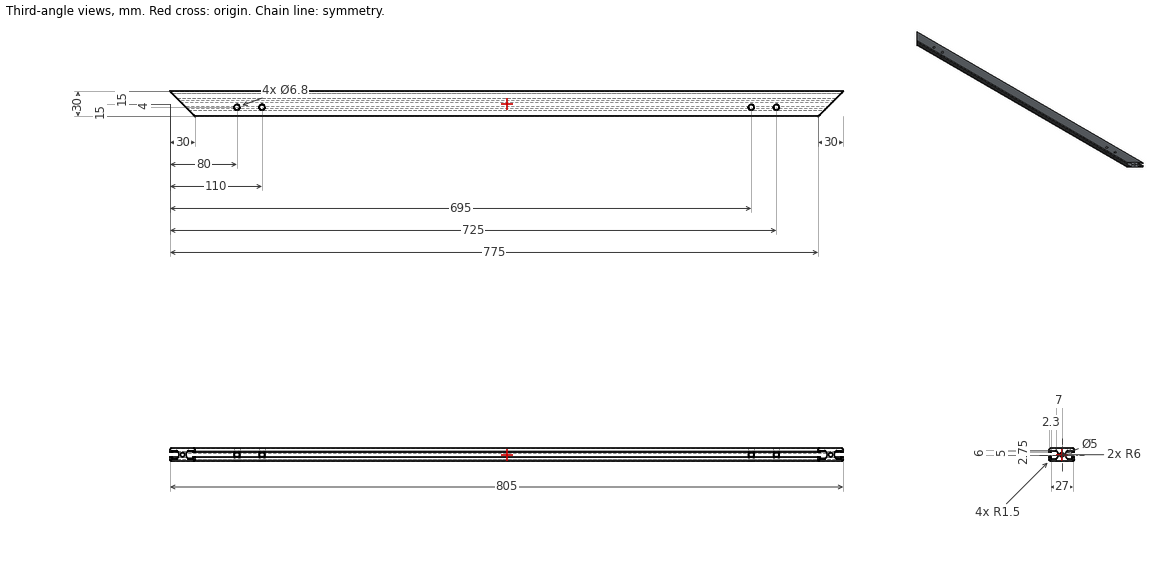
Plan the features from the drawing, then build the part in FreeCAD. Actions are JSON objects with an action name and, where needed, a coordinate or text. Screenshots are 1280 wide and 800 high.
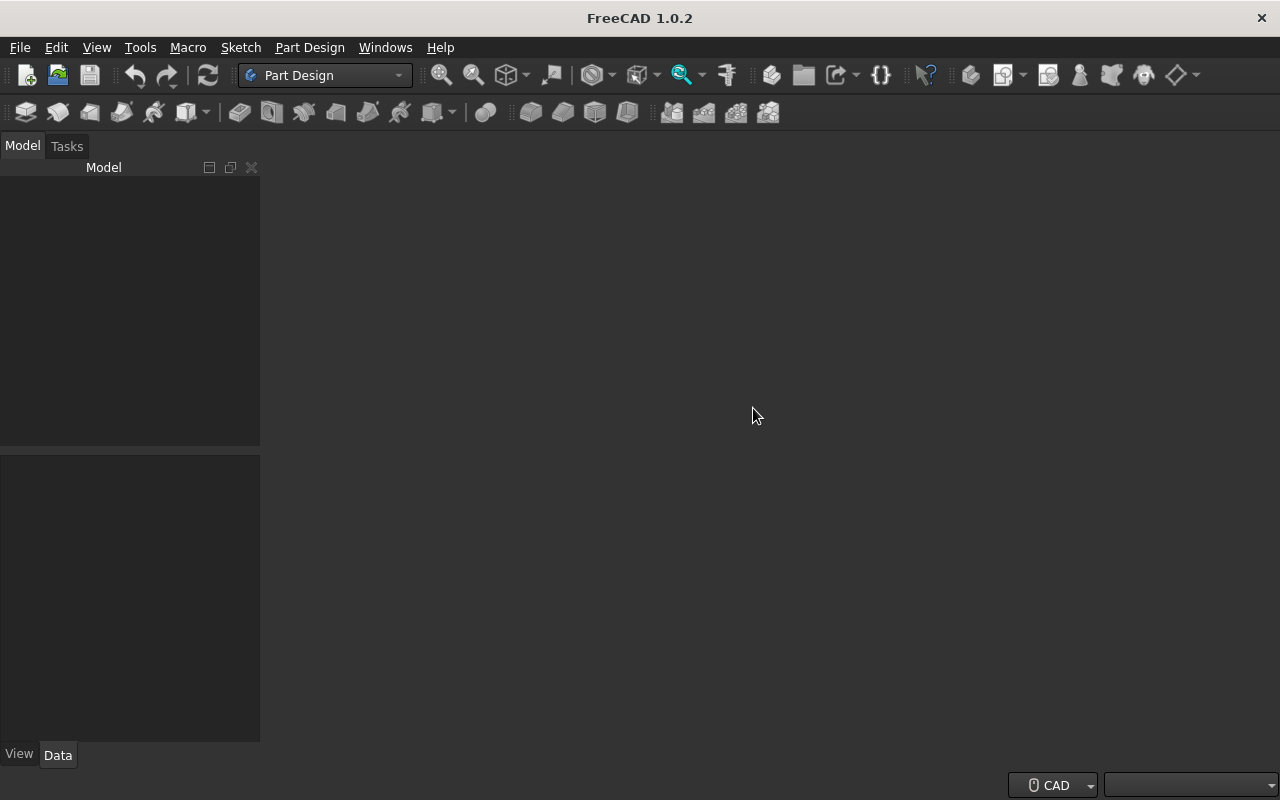
{"action": "left_click", "coordinate": [26, 76]}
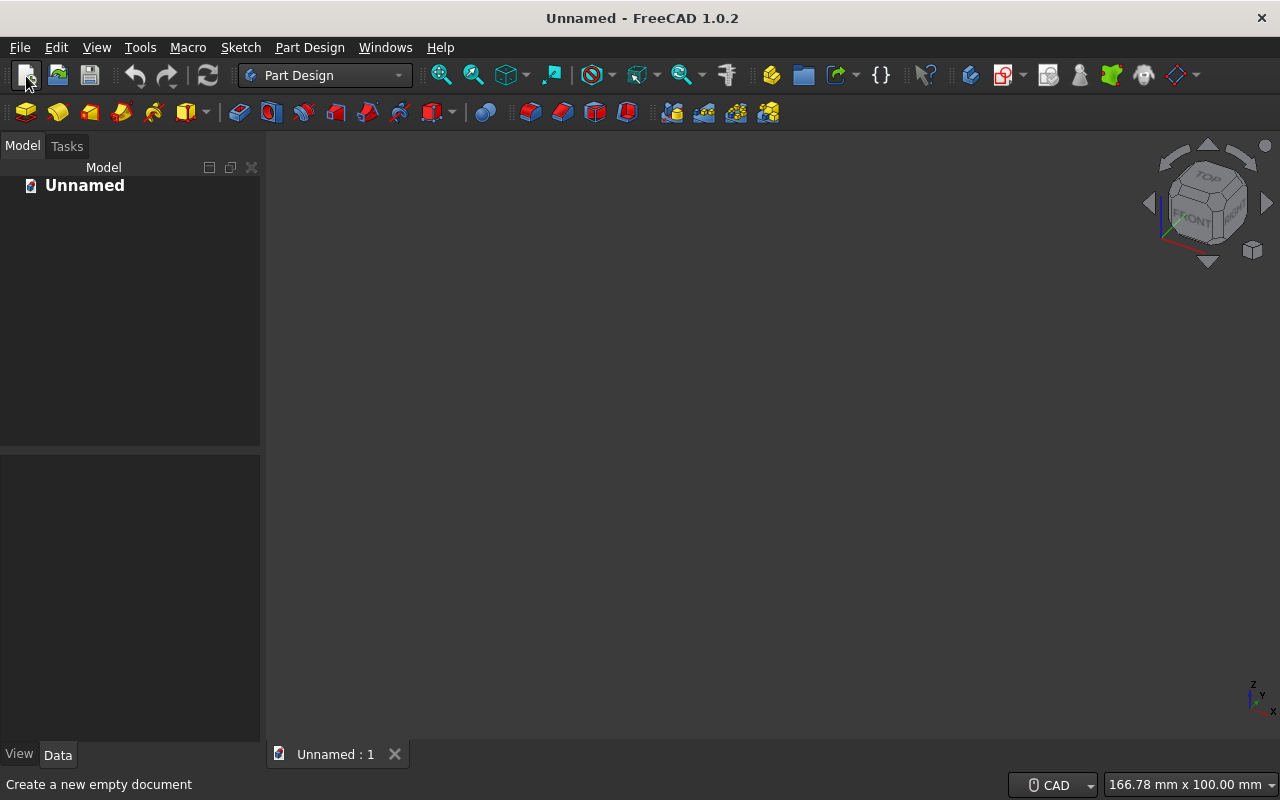
{"action": "left_click", "coordinate": [972, 76]}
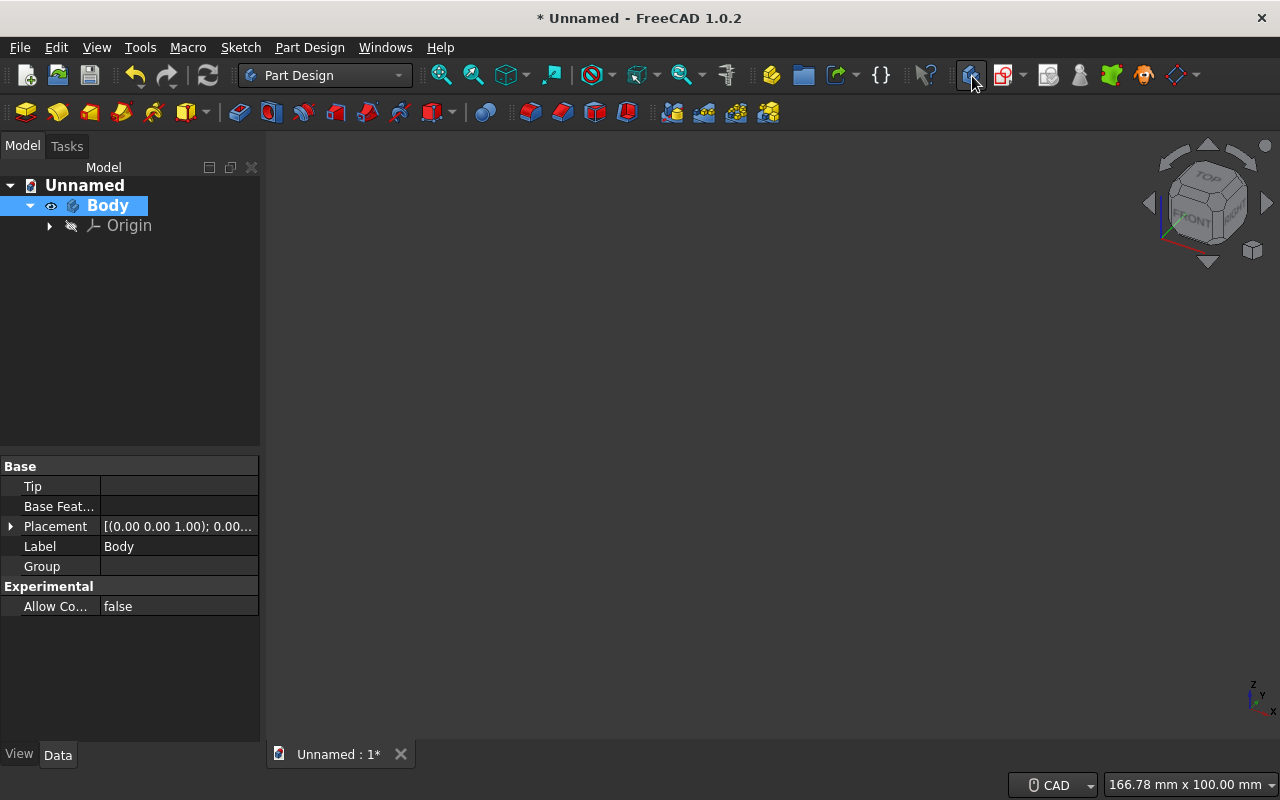
{"action": "left_click", "coordinate": [50, 226]}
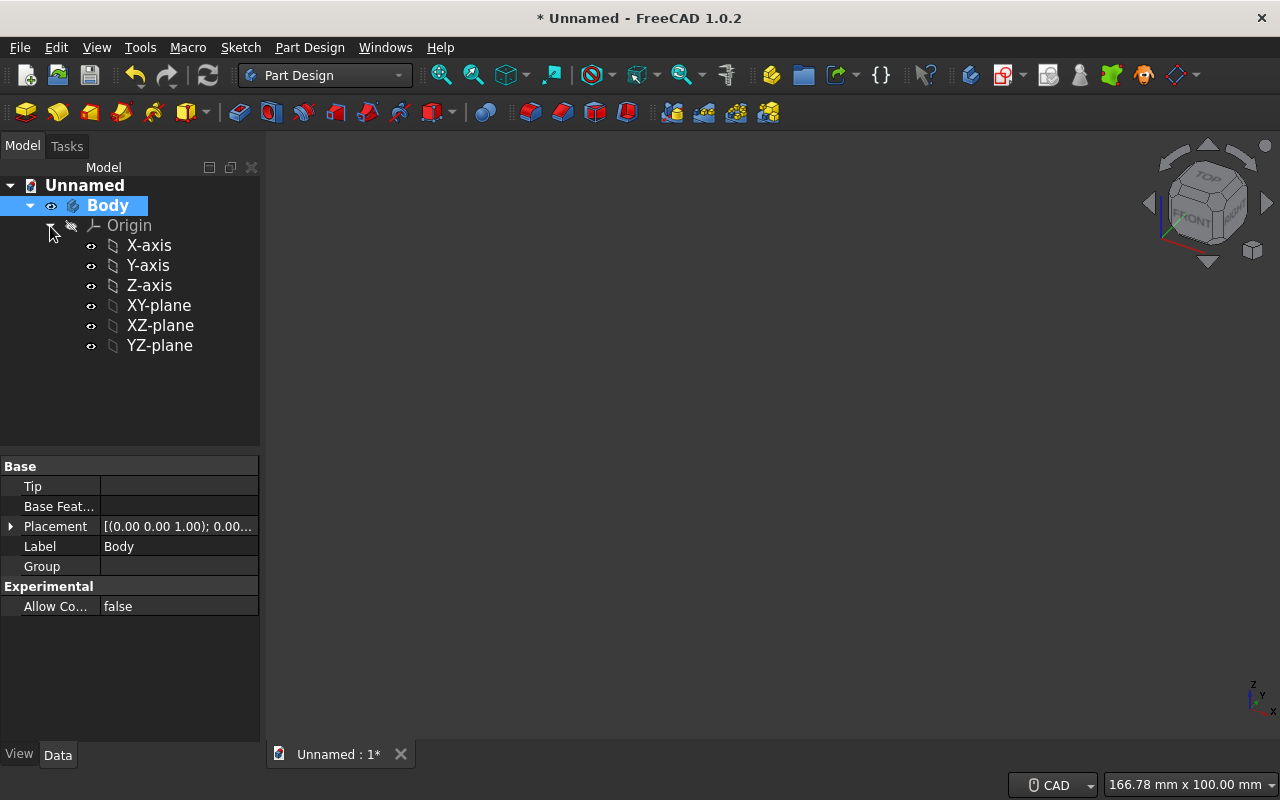
{"action": "left_click", "coordinate": [136, 346]}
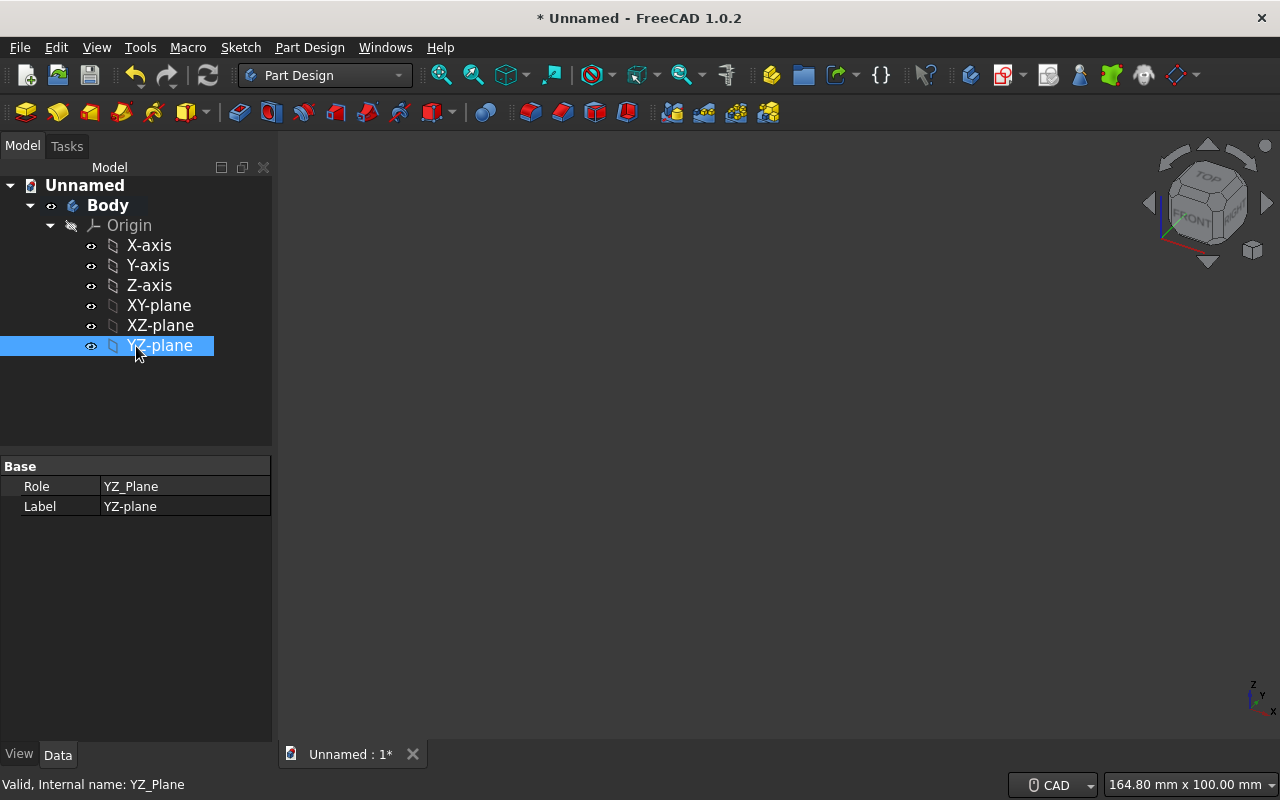
{"action": "left_click", "coordinate": [1176, 76]}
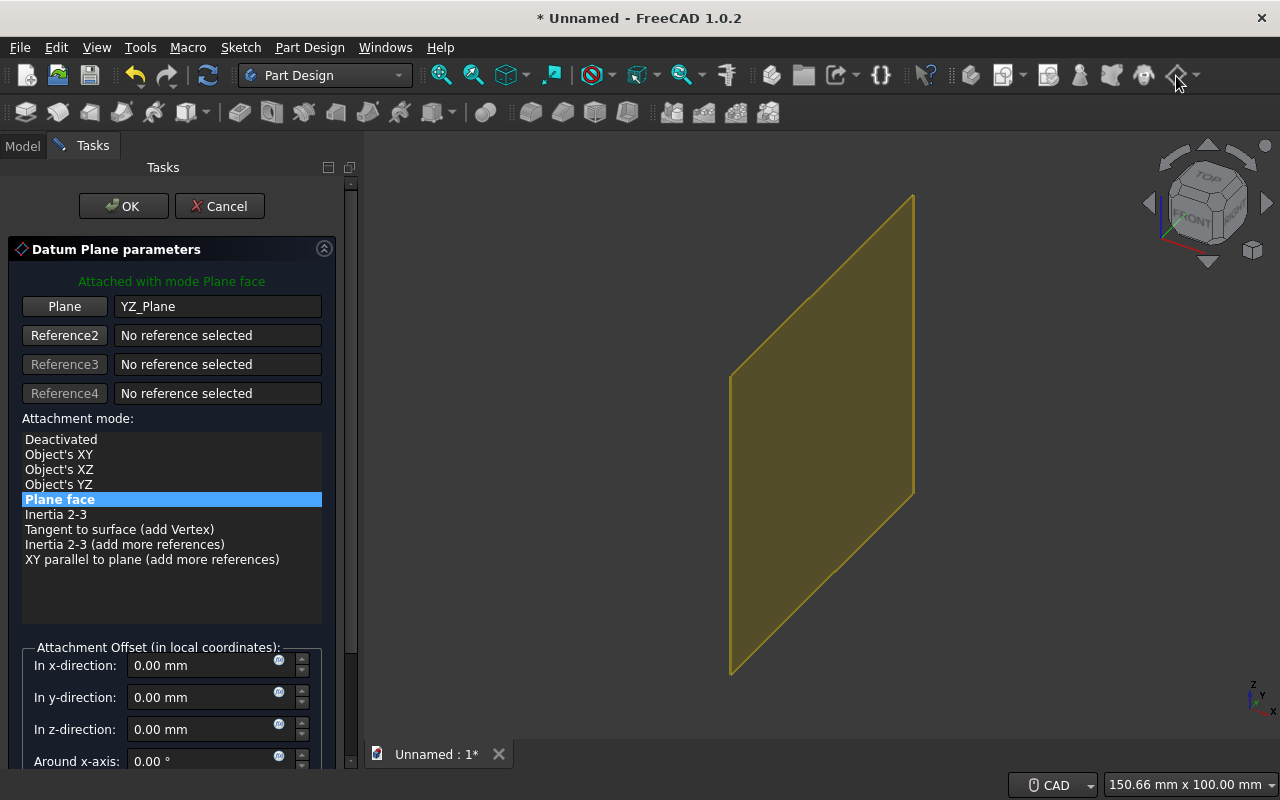
{"action": "triple_click", "coordinate": [210, 729]}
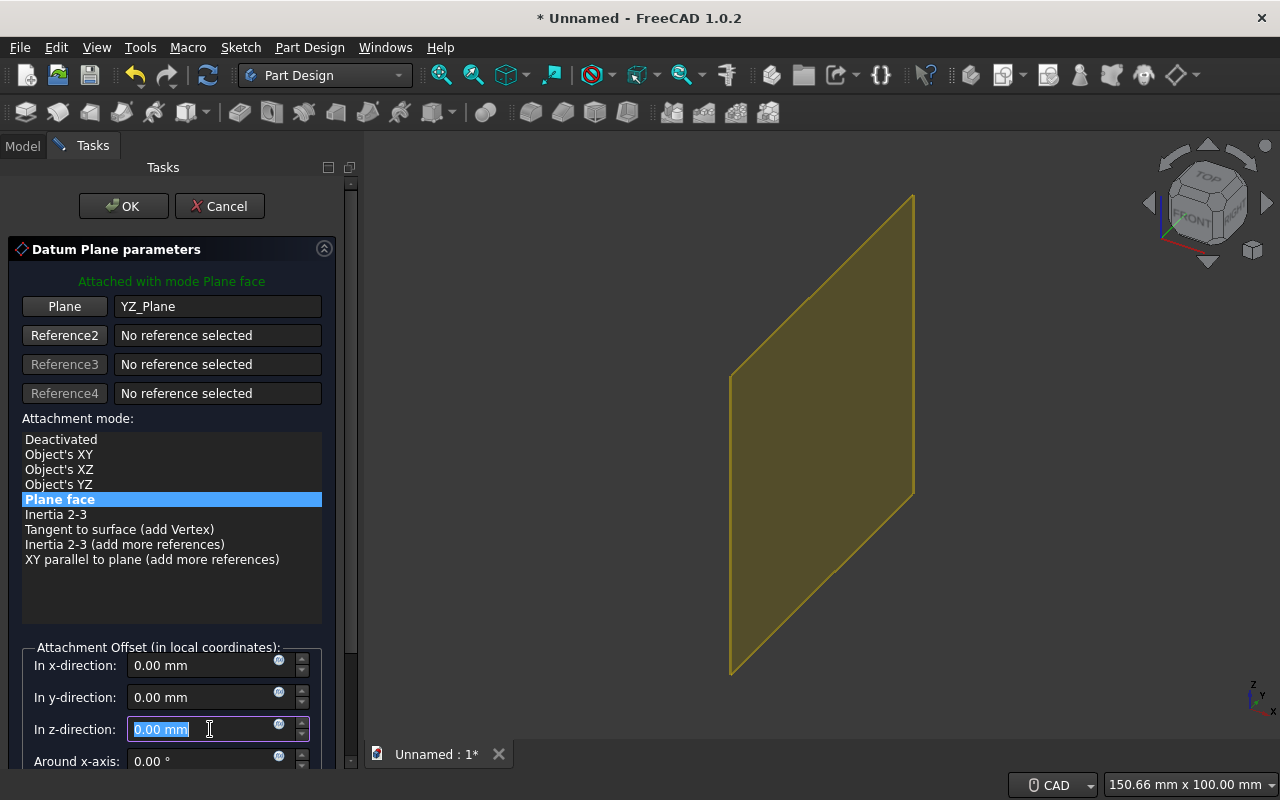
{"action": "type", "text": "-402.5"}
{"action": "key", "text": "Tab"}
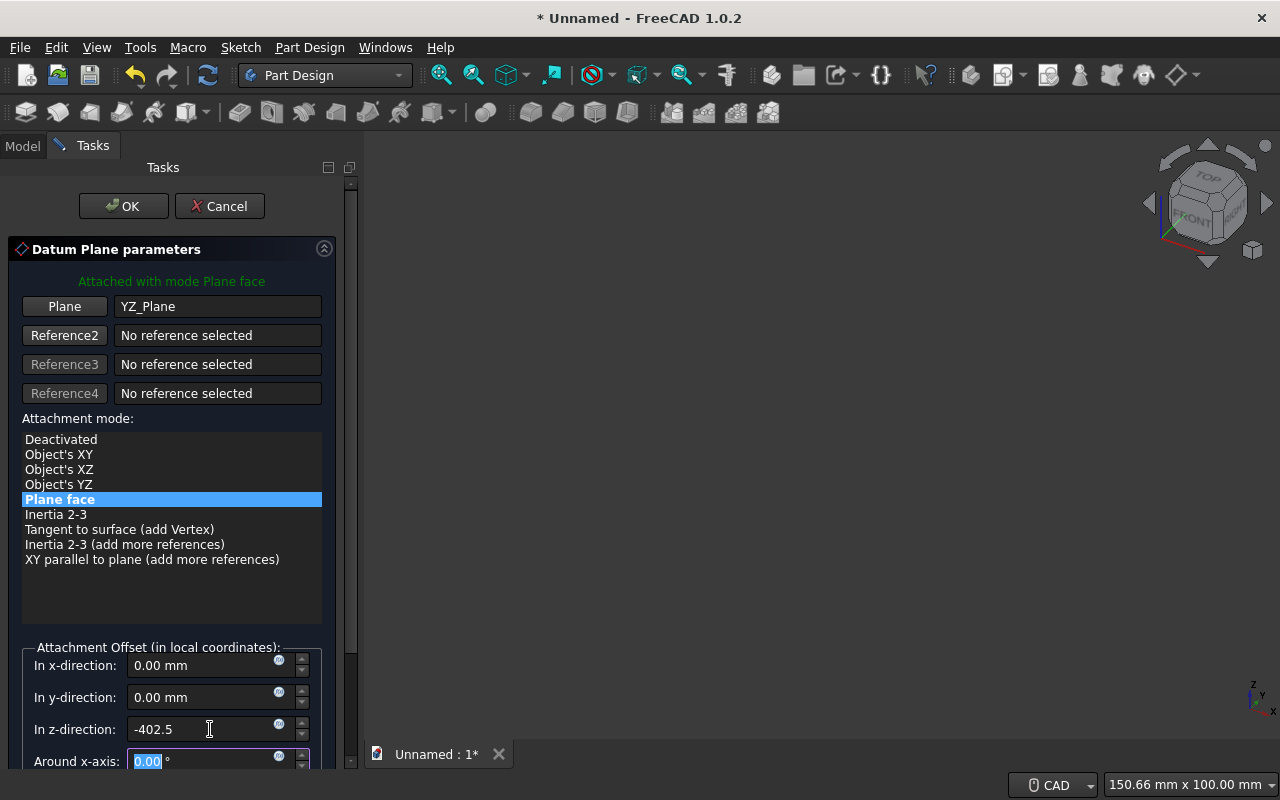
{"action": "left_click", "coordinate": [124, 206]}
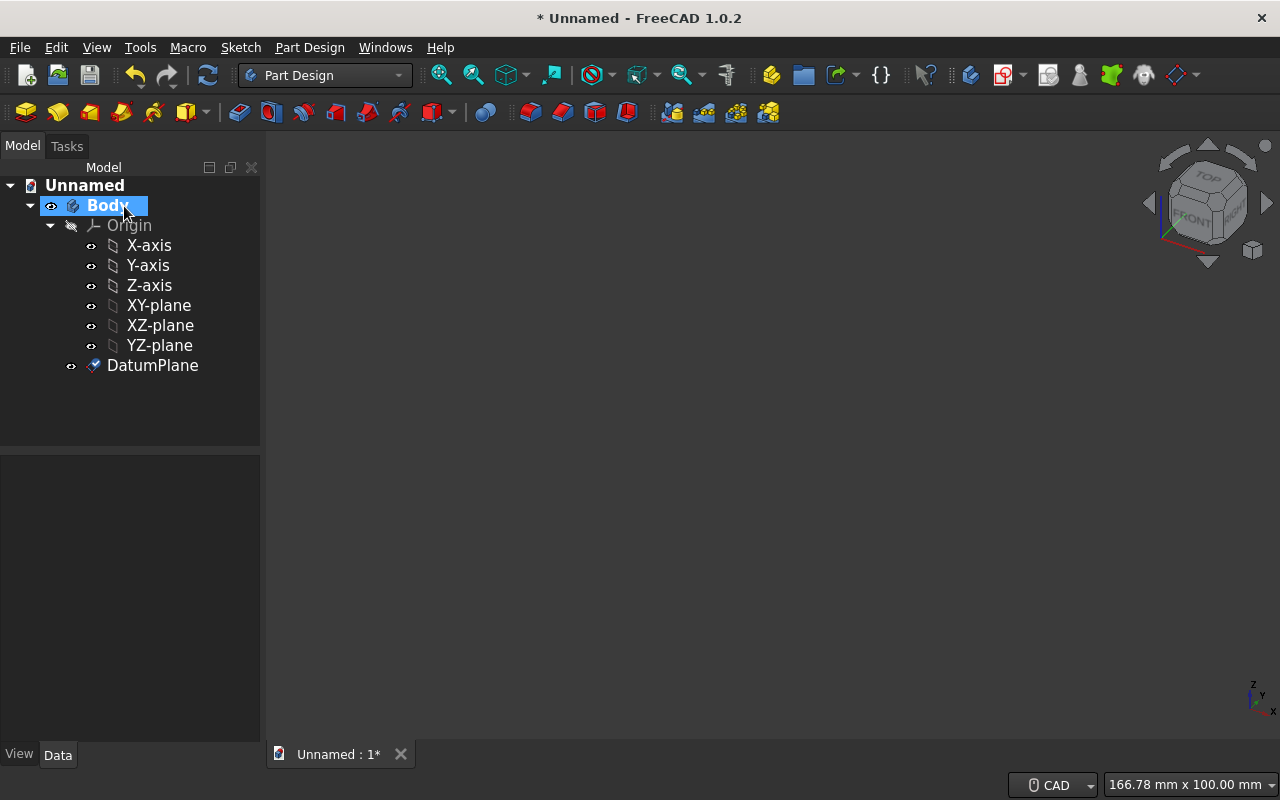
{"action": "left_click", "coordinate": [116, 366]}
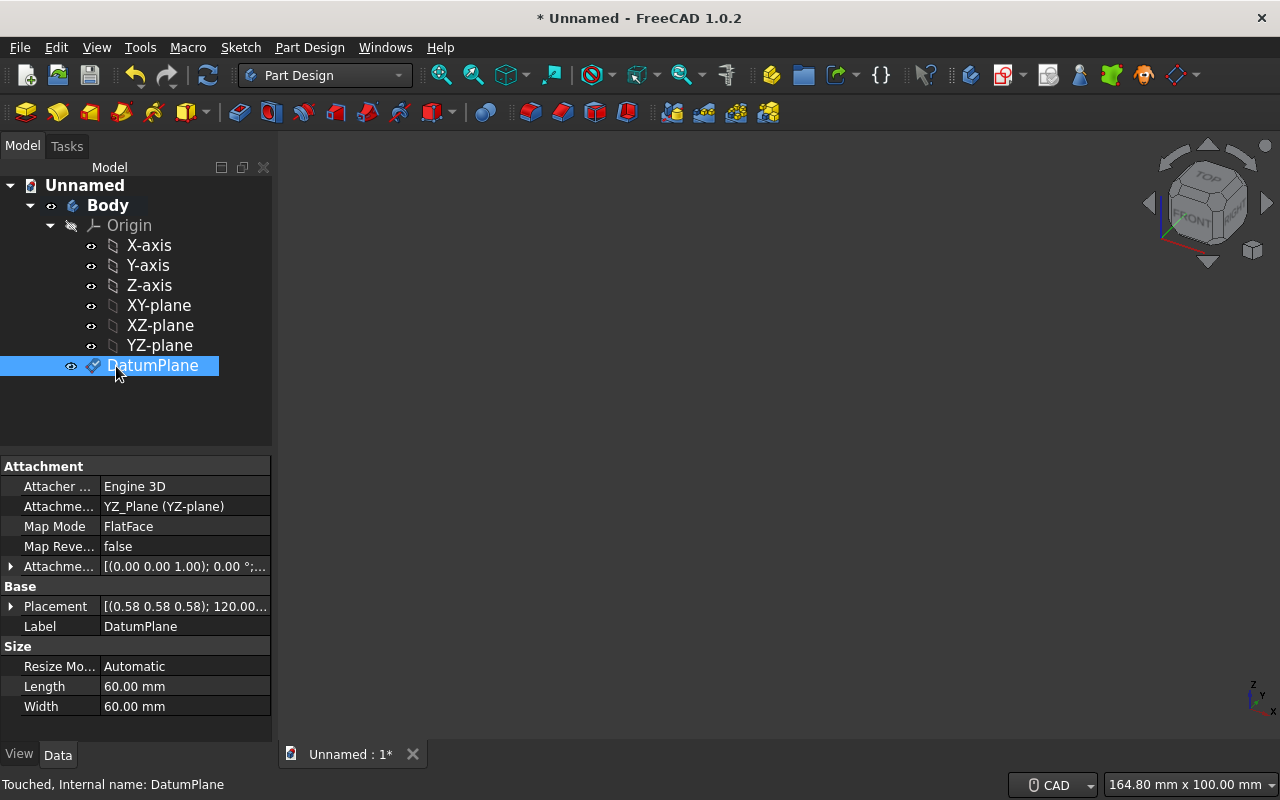
{"action": "left_click", "coordinate": [1004, 76]}